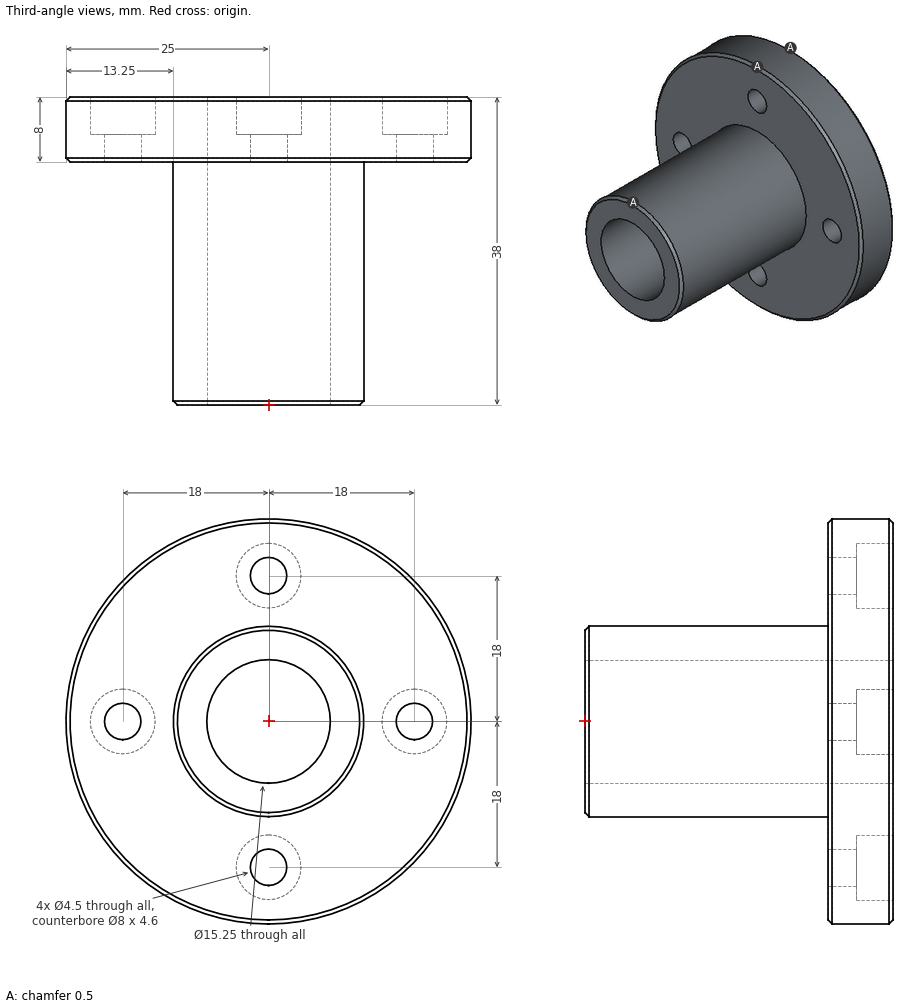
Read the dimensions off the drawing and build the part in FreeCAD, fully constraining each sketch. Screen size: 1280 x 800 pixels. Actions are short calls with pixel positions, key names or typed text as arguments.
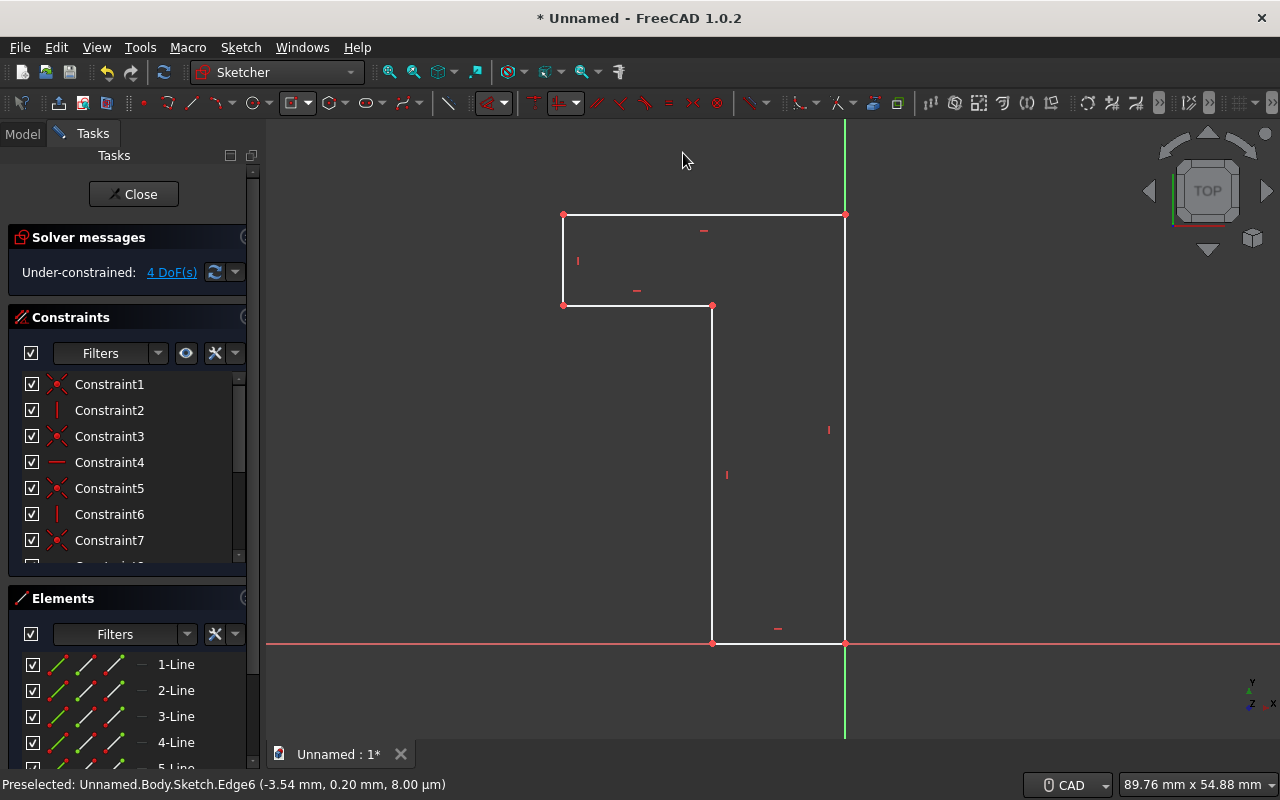
click(488, 104)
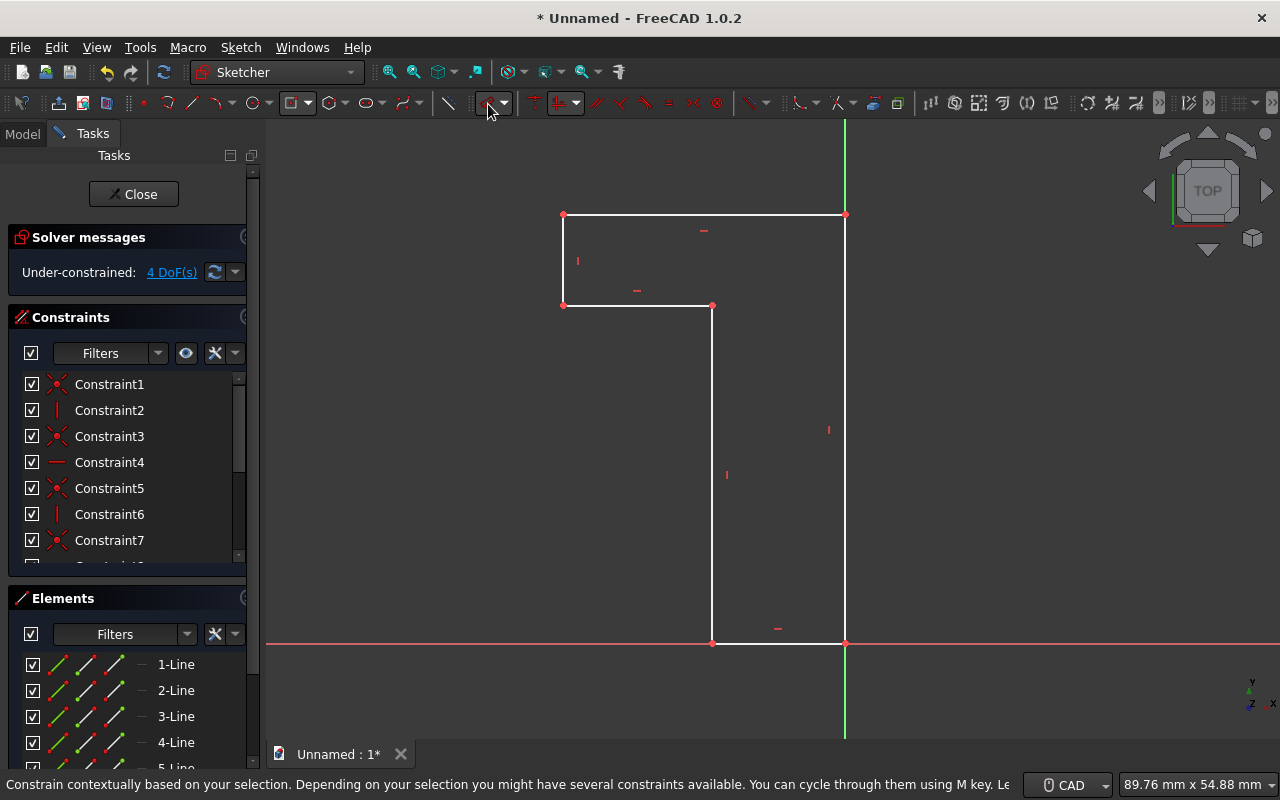
click(563, 242)
click(529, 260)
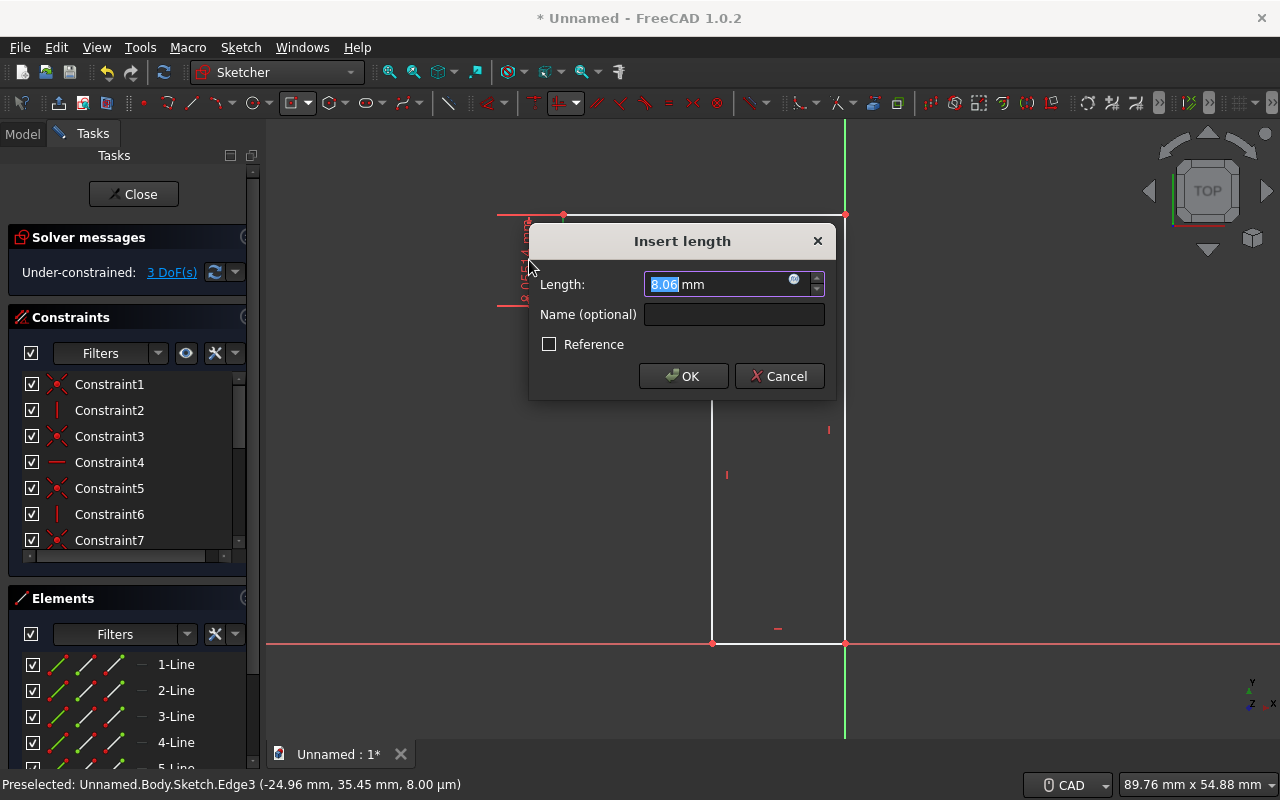
text(8)
key(Return)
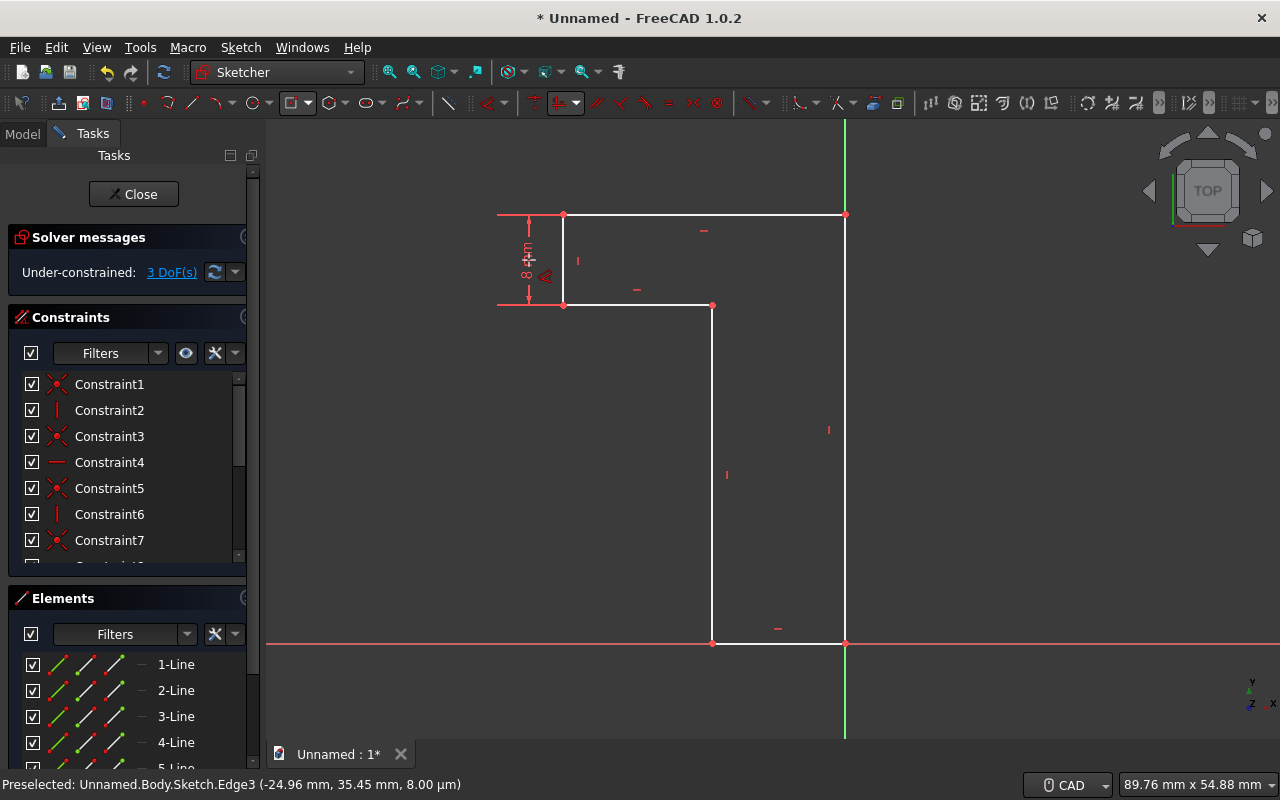
click(845, 515)
click(879, 429)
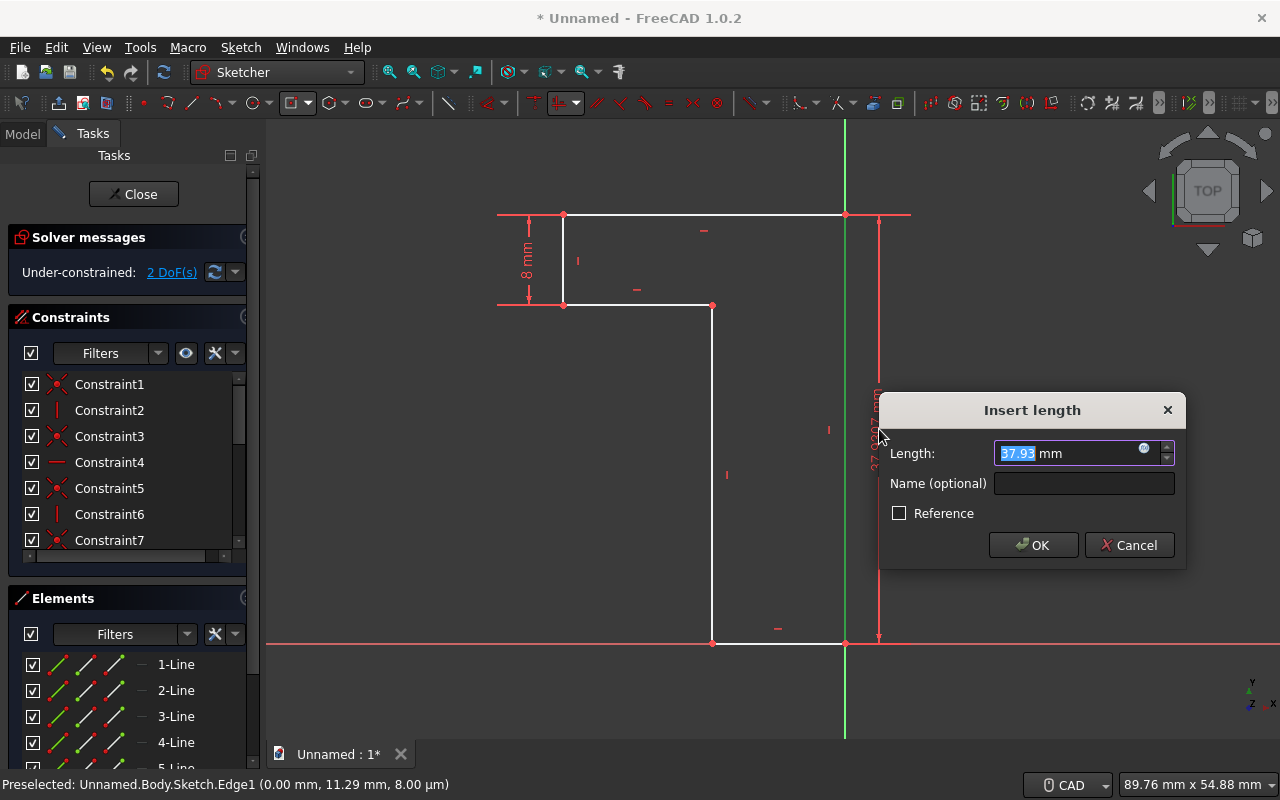
text(38)
key(Return)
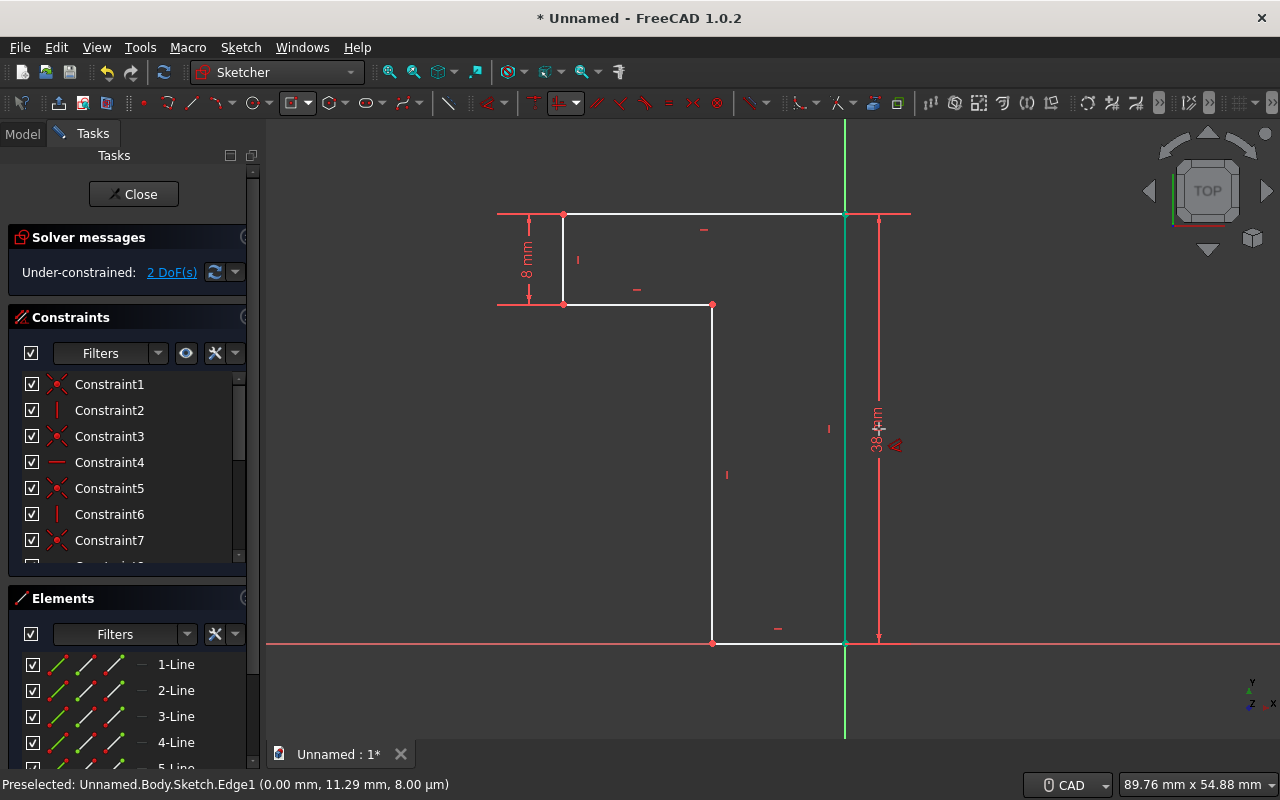
click(760, 214)
click(704, 180)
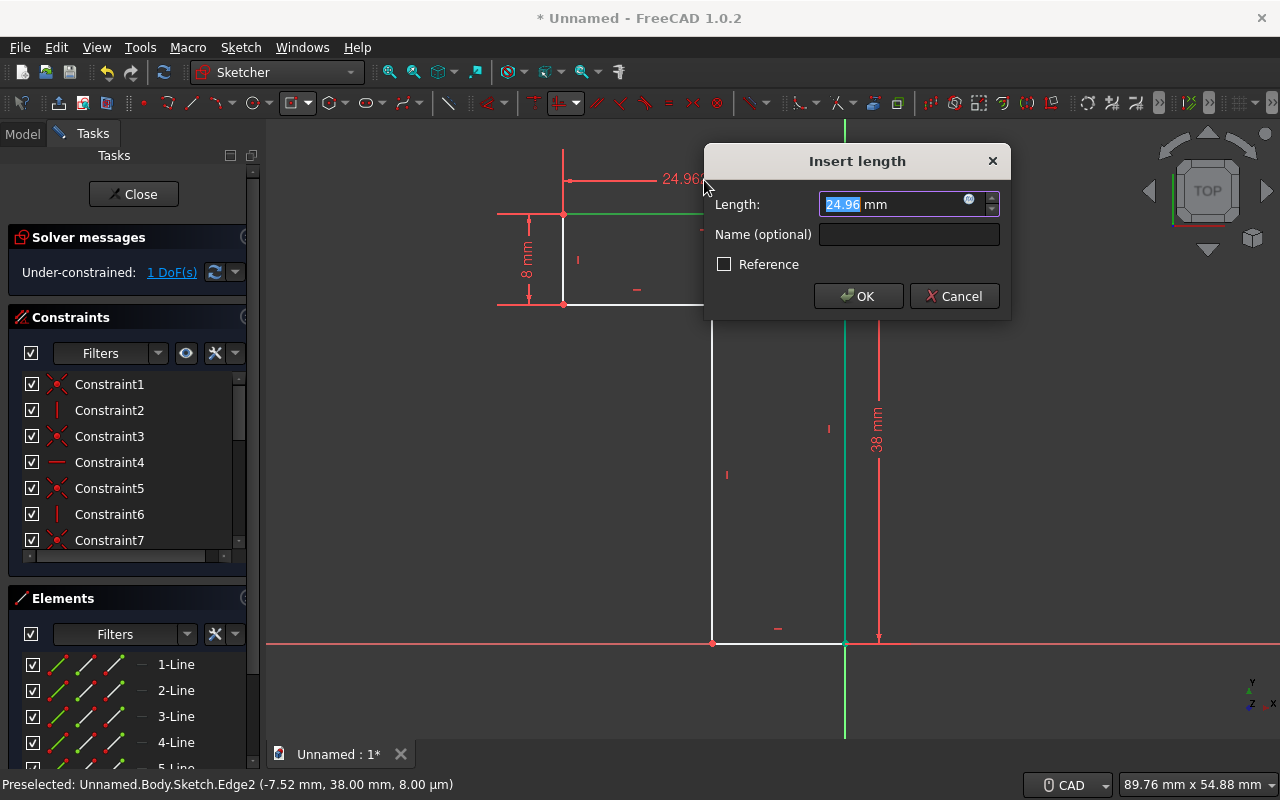
text(25)
key(Return)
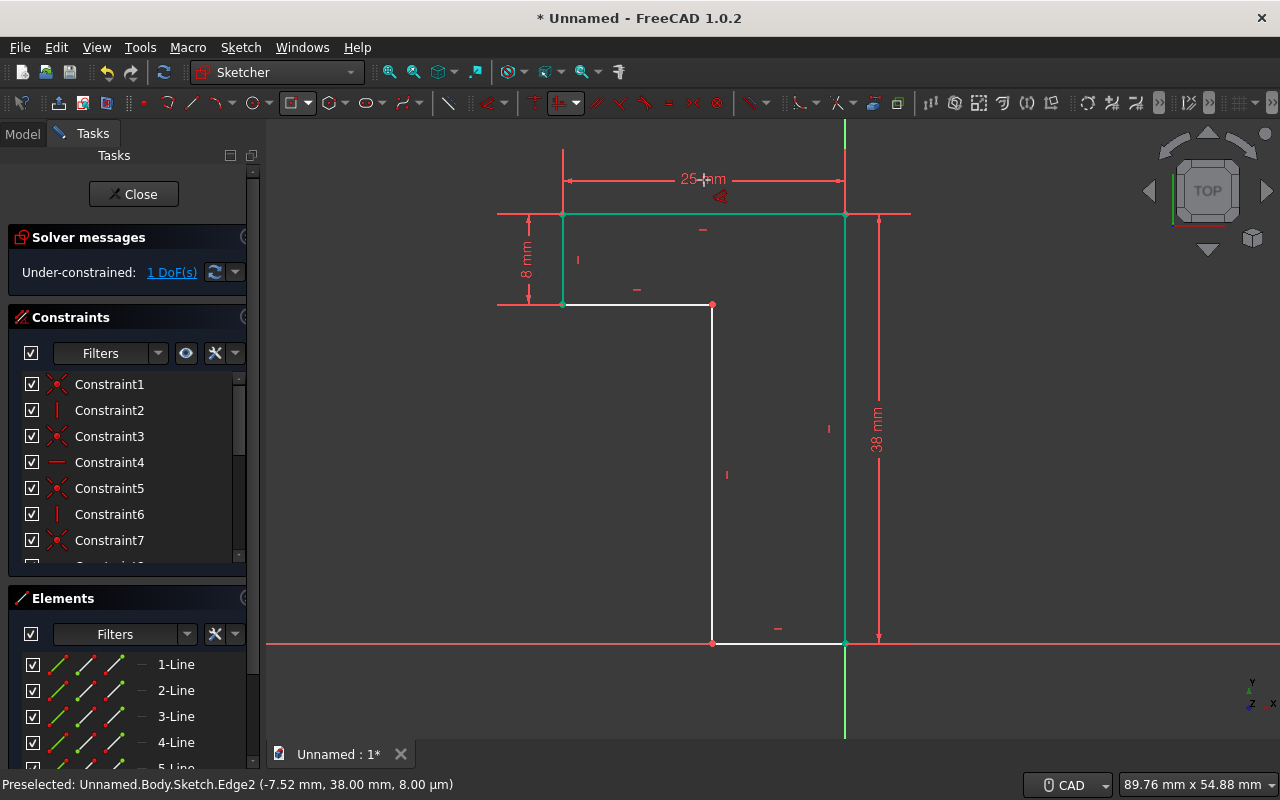
click(607, 305)
click(637, 271)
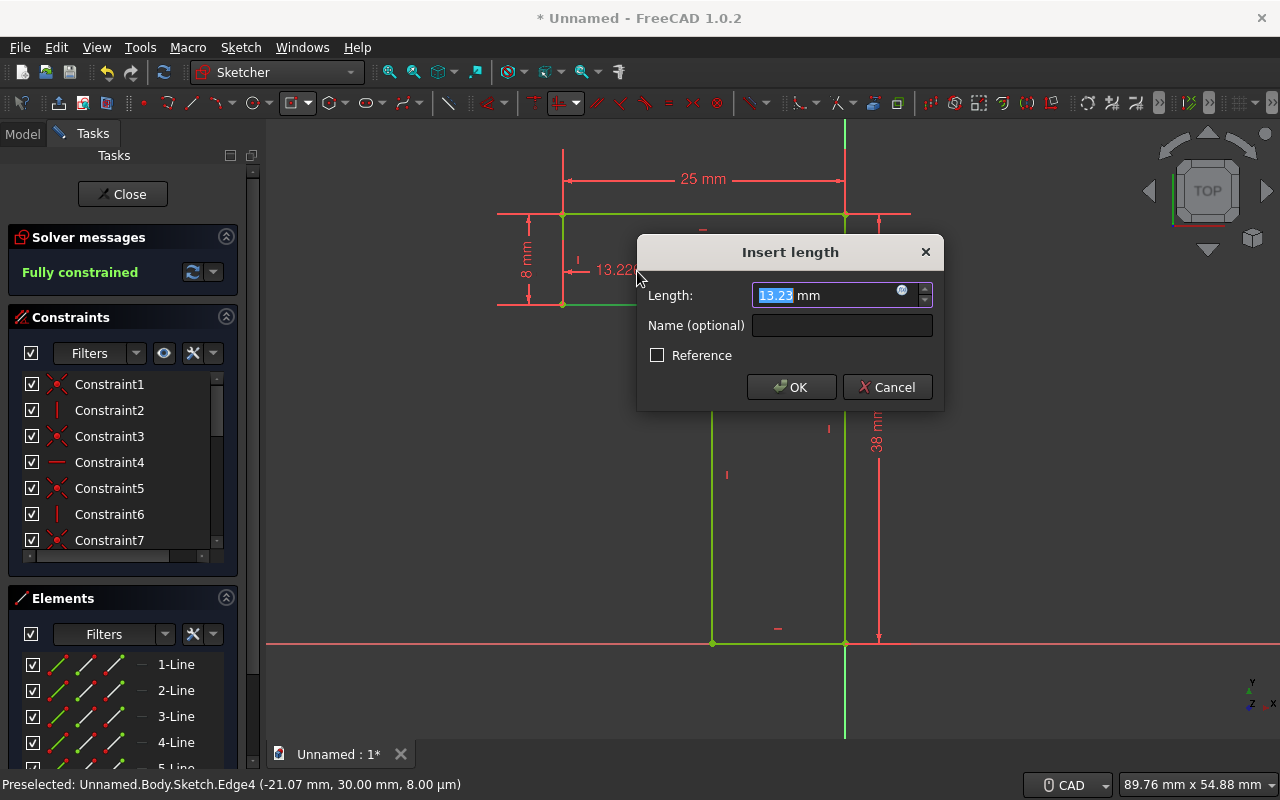
text(13.25)
key(Return)
key(Escape)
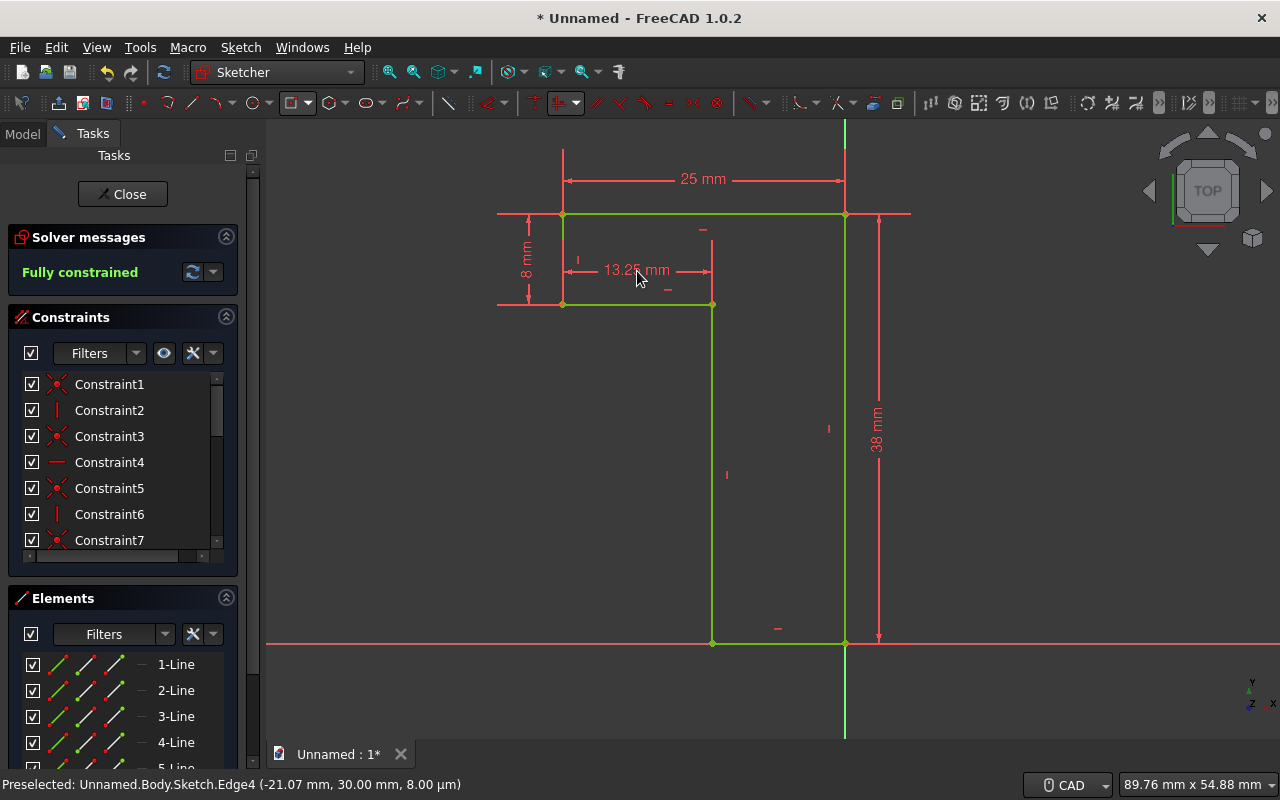
click(123, 194)